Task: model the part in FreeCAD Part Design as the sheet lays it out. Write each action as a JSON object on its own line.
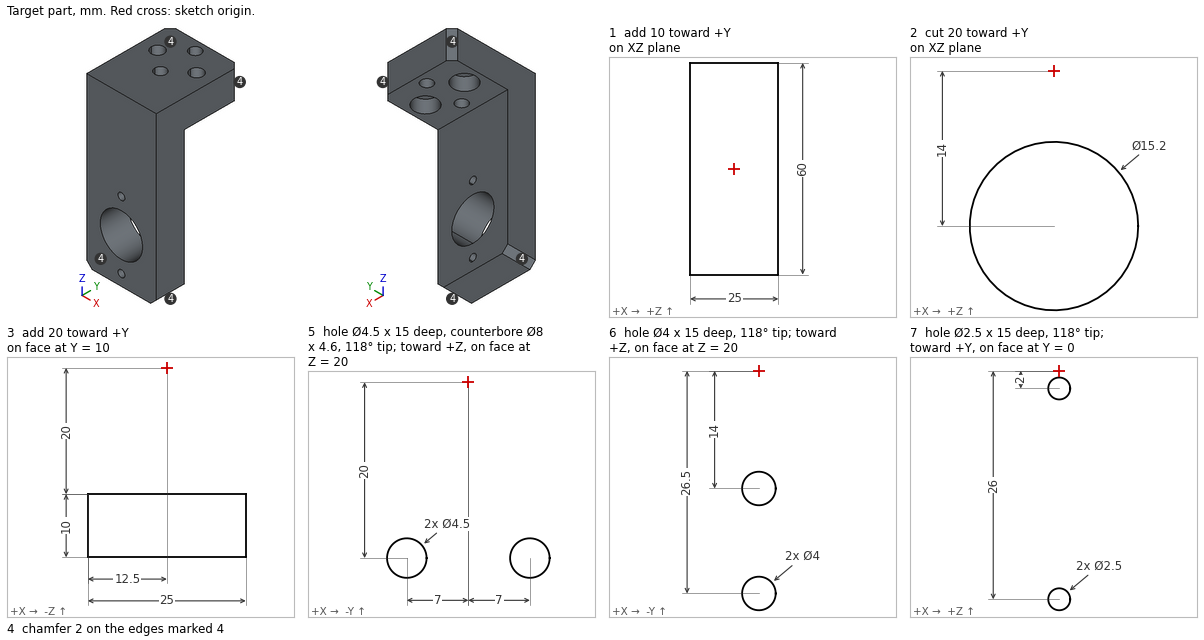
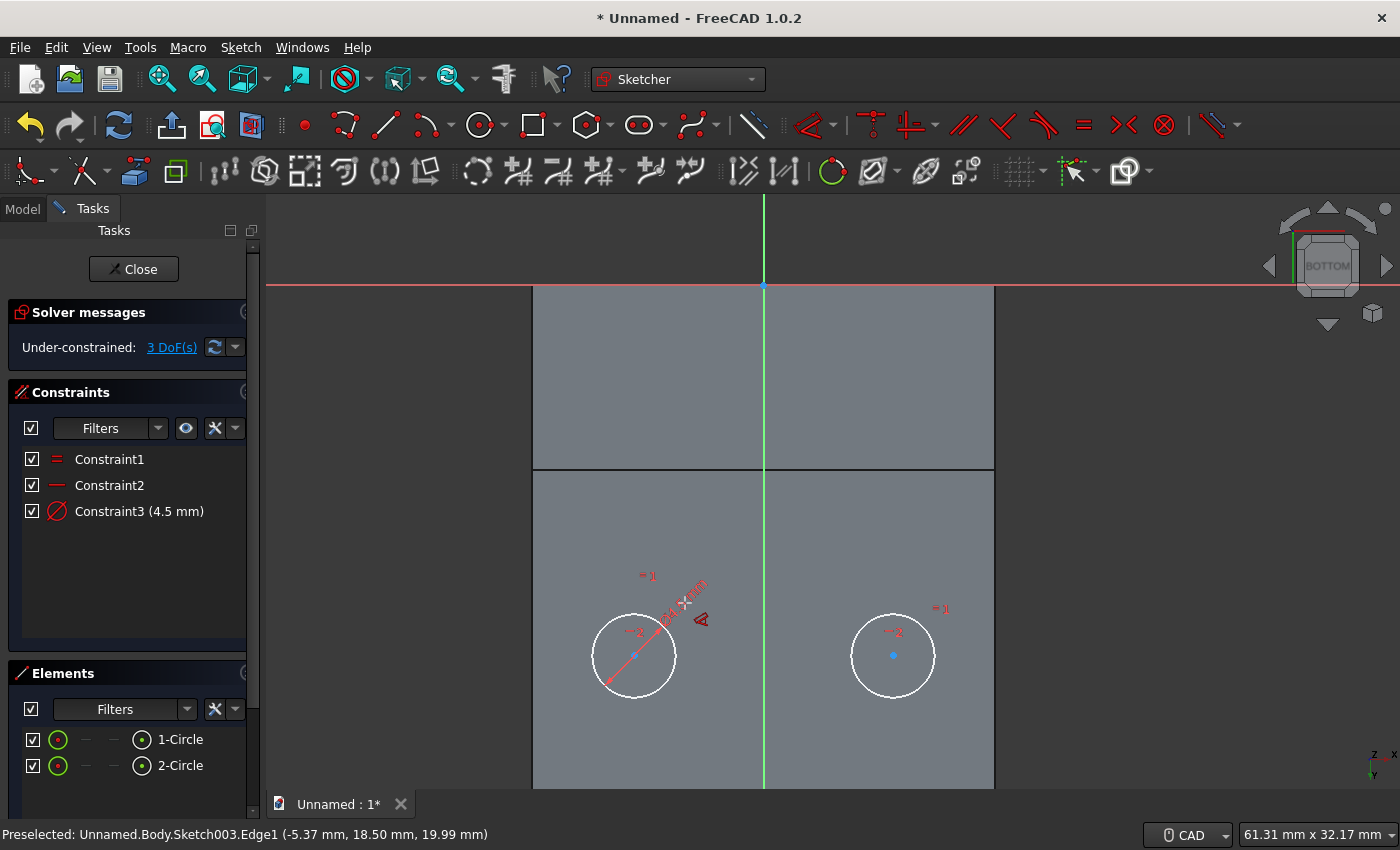
{"action": "left_click", "coordinate": [634, 656]}
{"action": "left_click", "coordinate": [699, 251]}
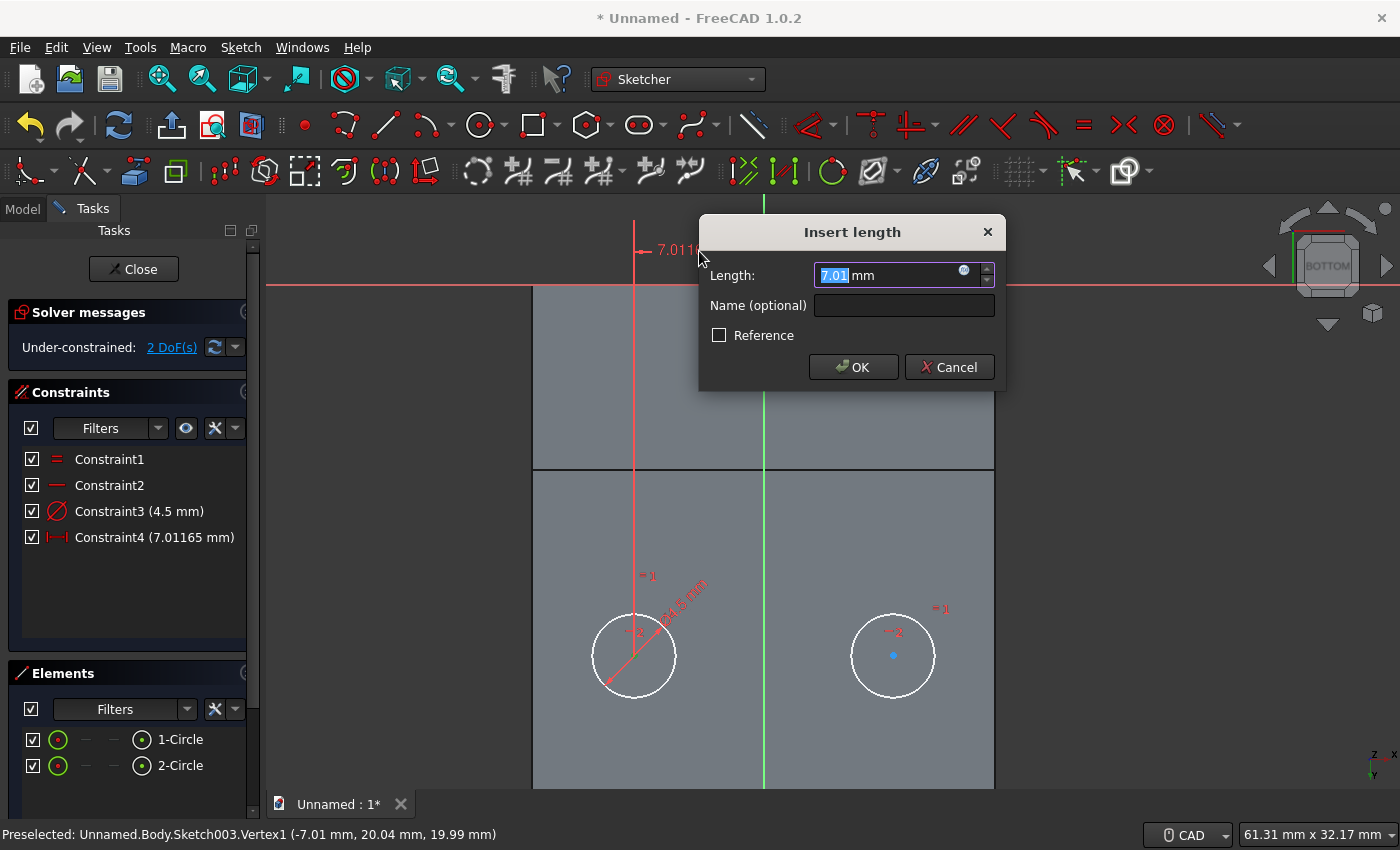
{"action": "type", "text": "7"}
{"action": "key", "text": "Return"}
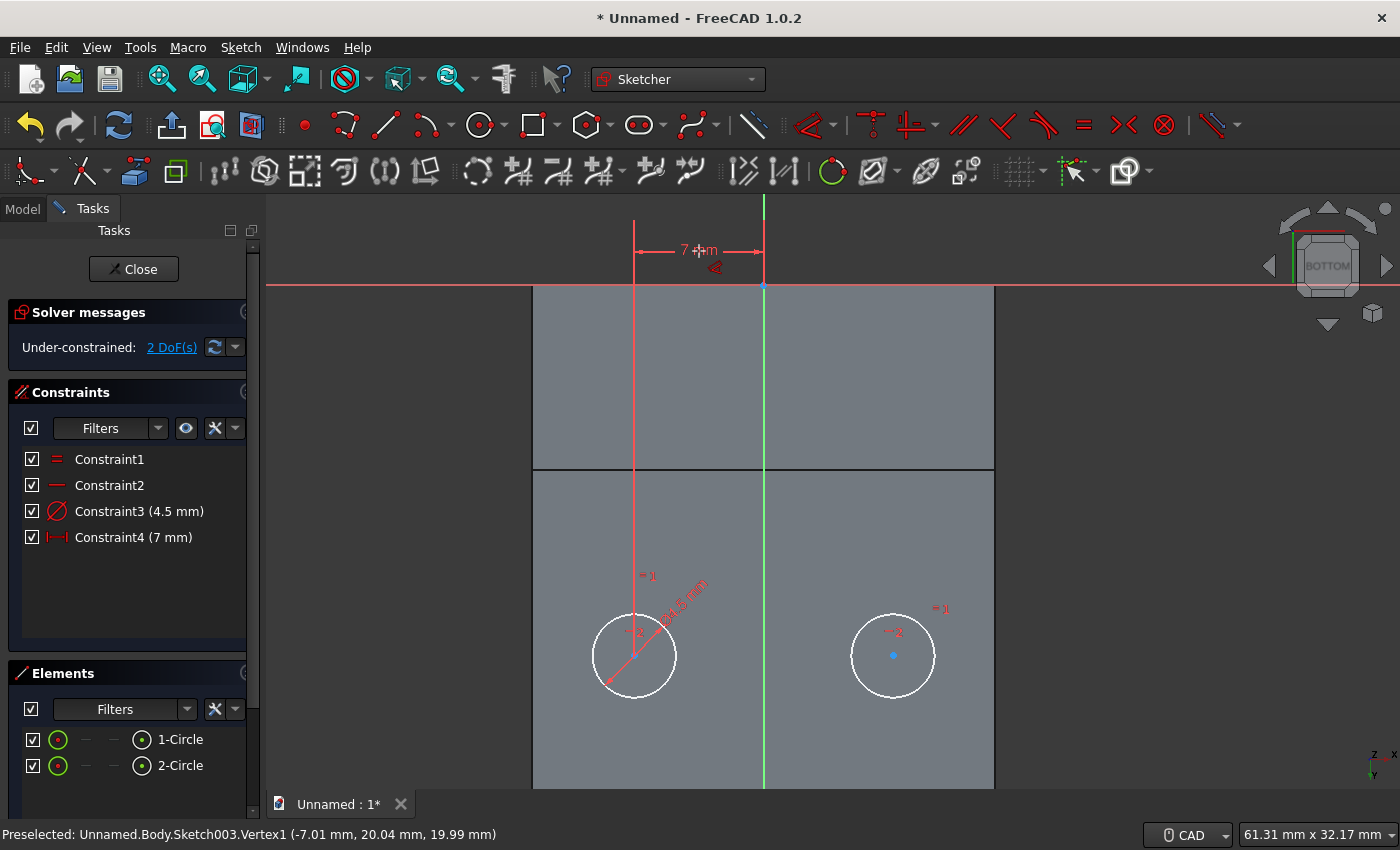
{"action": "left_click", "coordinate": [893, 656]}
{"action": "left_click", "coordinate": [828, 251]}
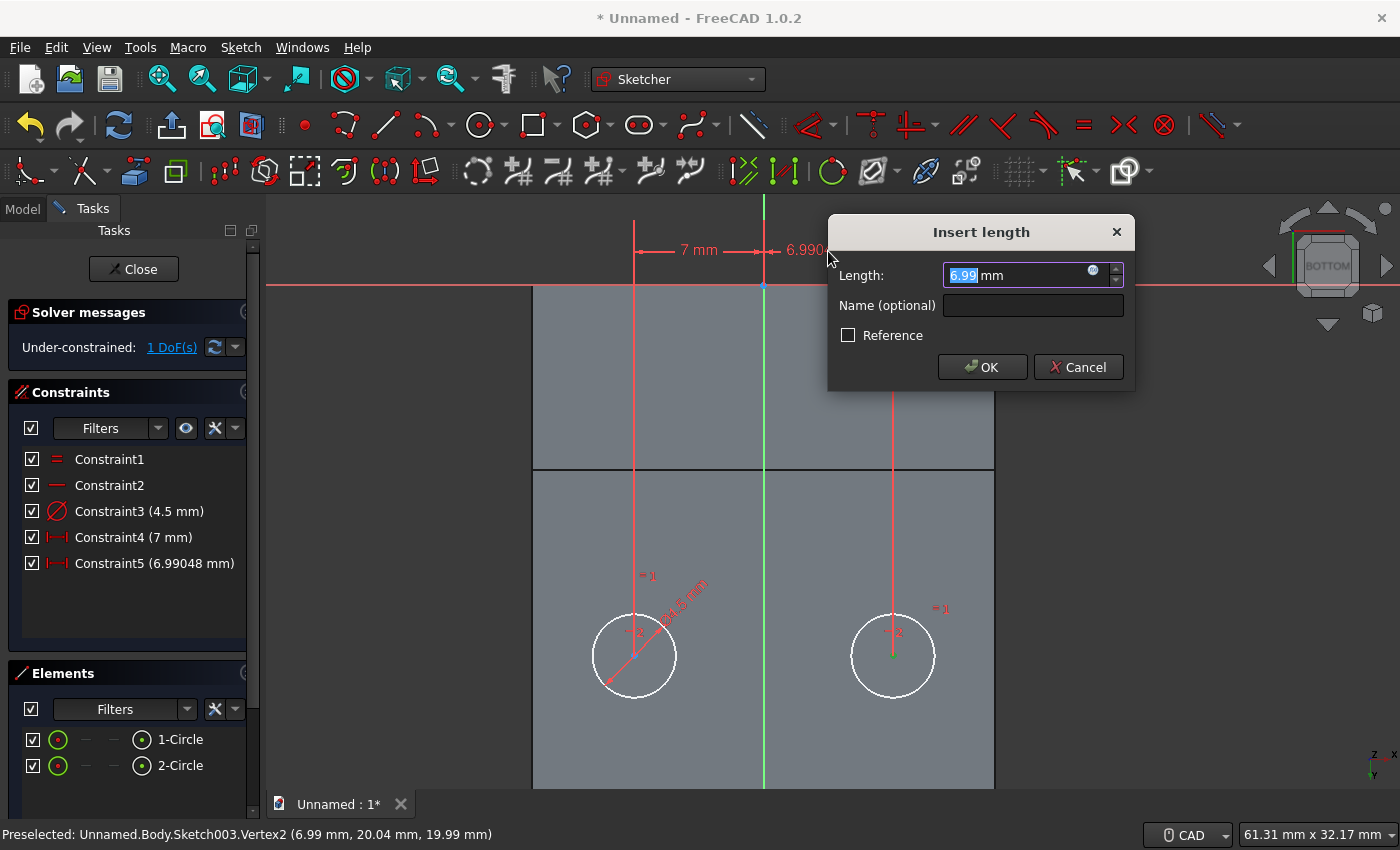
{"action": "type", "text": "7"}
{"action": "key", "text": "Return"}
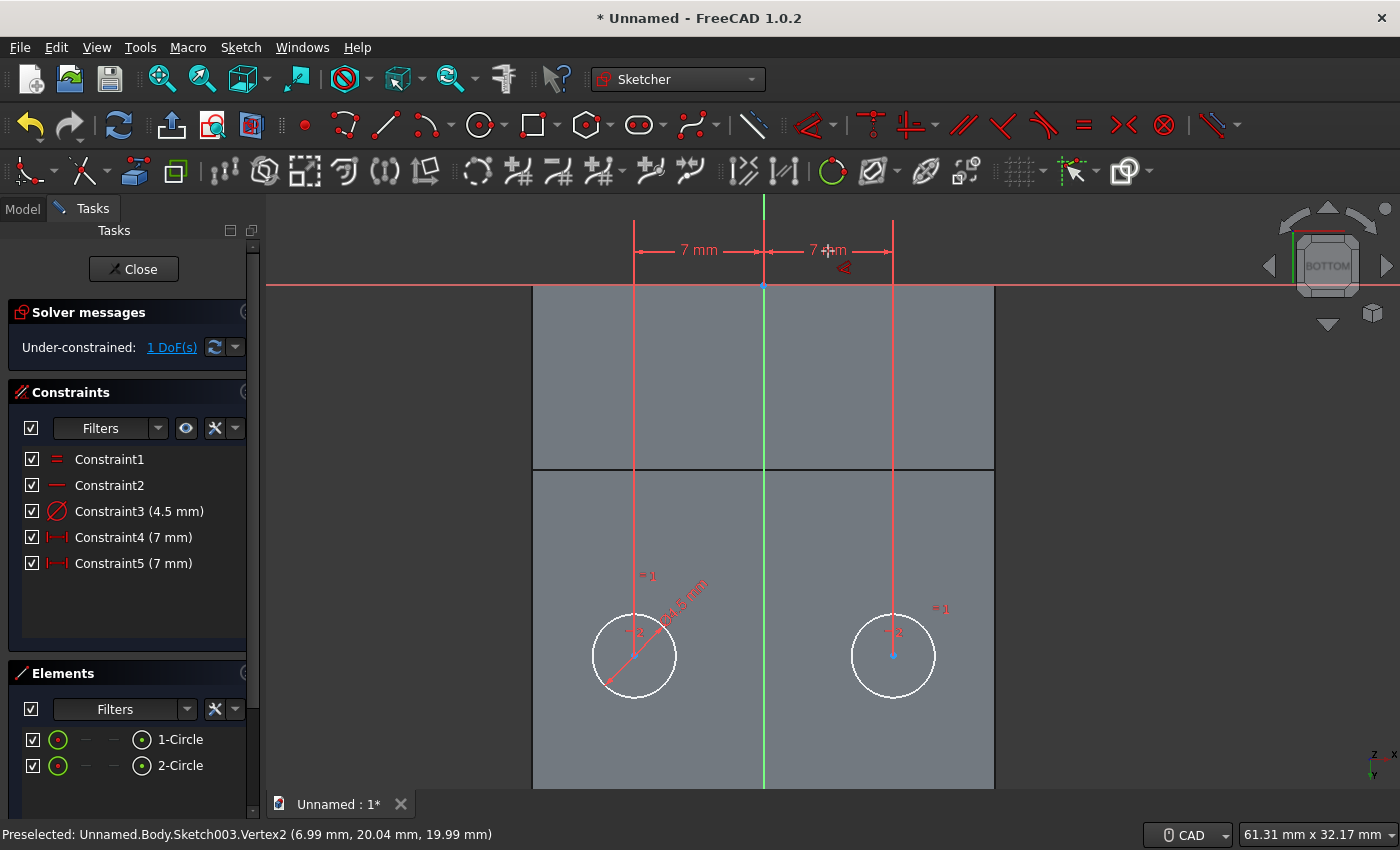
{"action": "left_click", "coordinate": [634, 656]}
{"action": "left_click", "coordinate": [600, 471]}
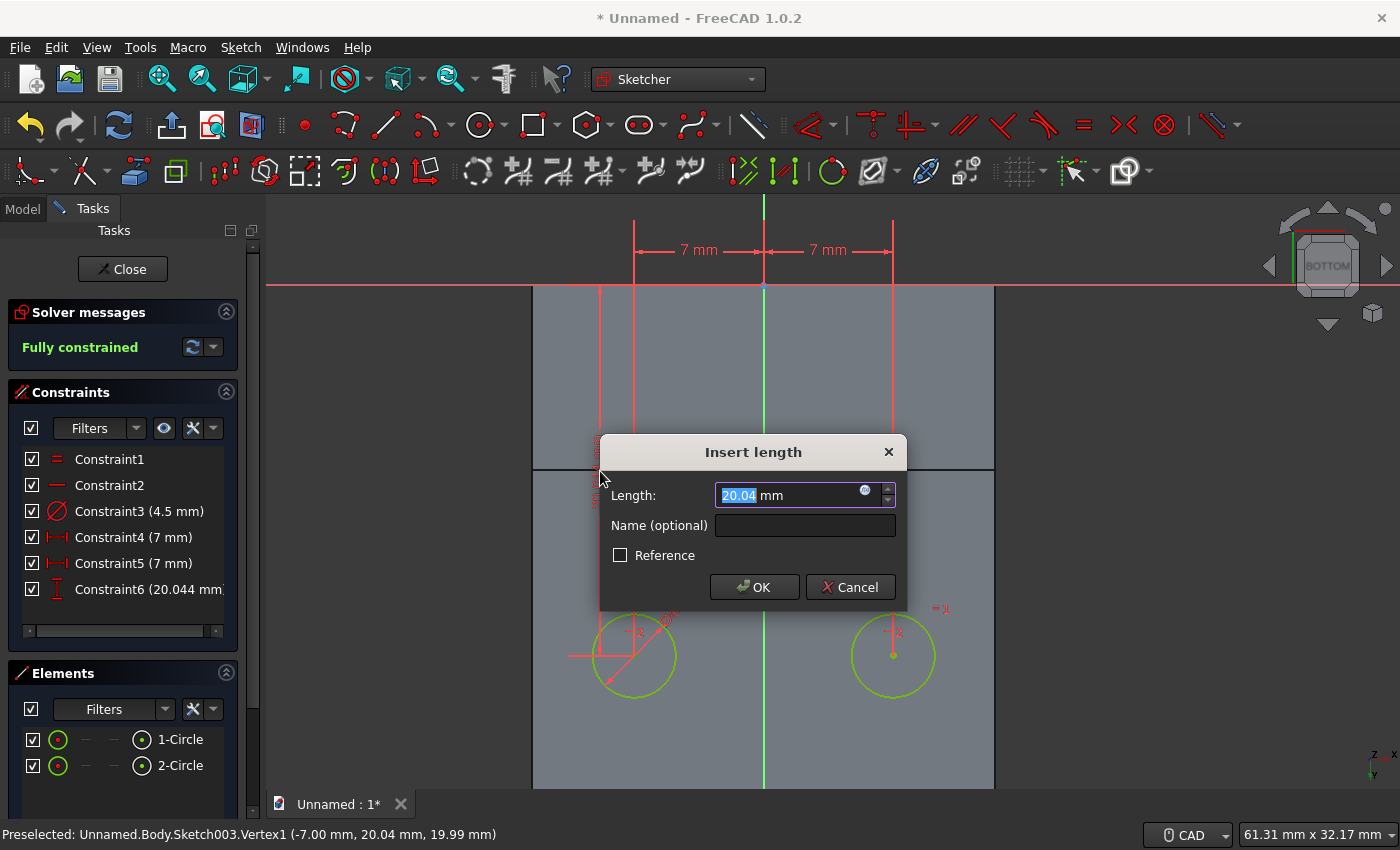
{"action": "type", "text": "20"}
{"action": "key", "text": "Return"}
{"action": "key", "text": "Escape"}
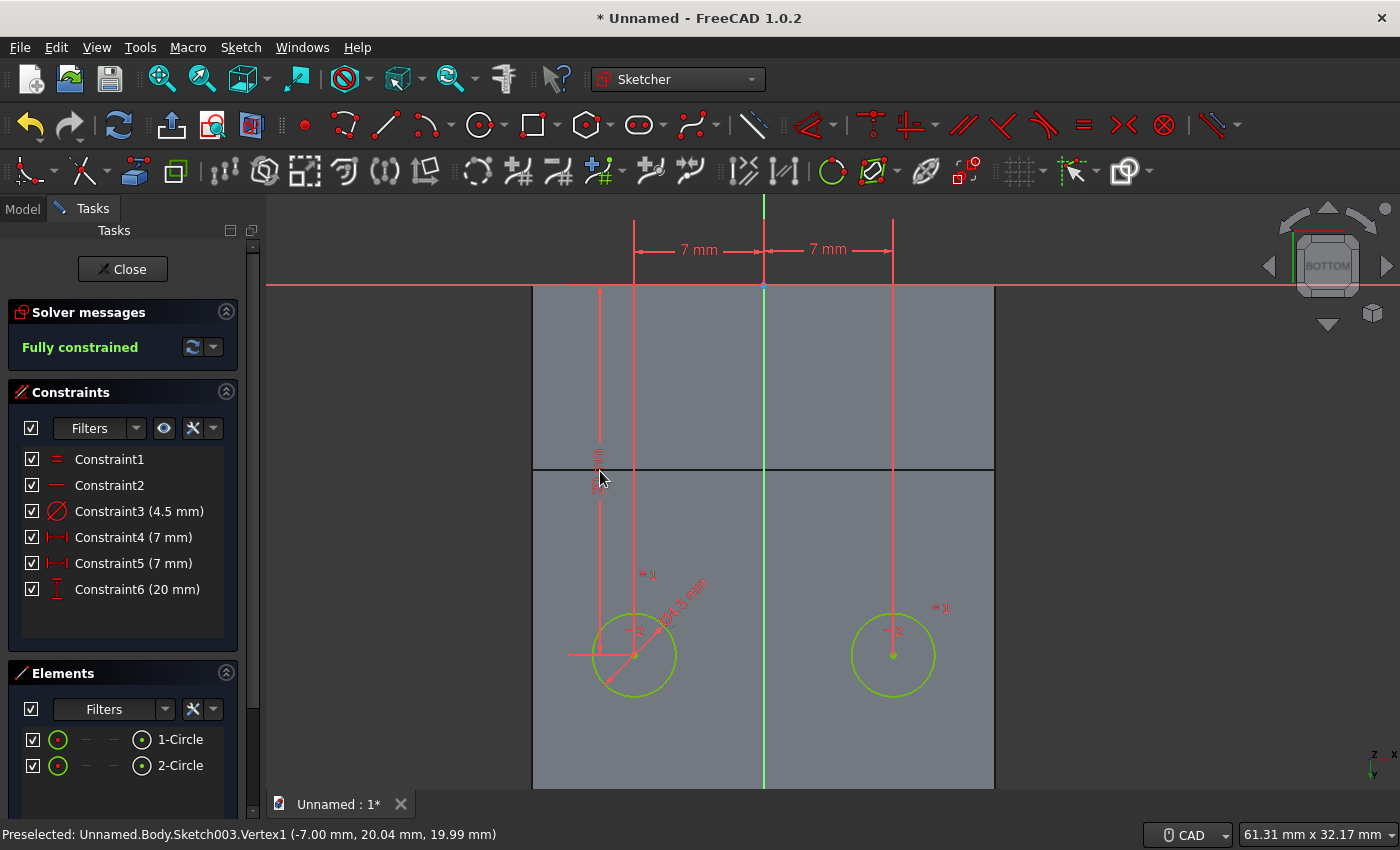
{"action": "left_click", "coordinate": [123, 269]}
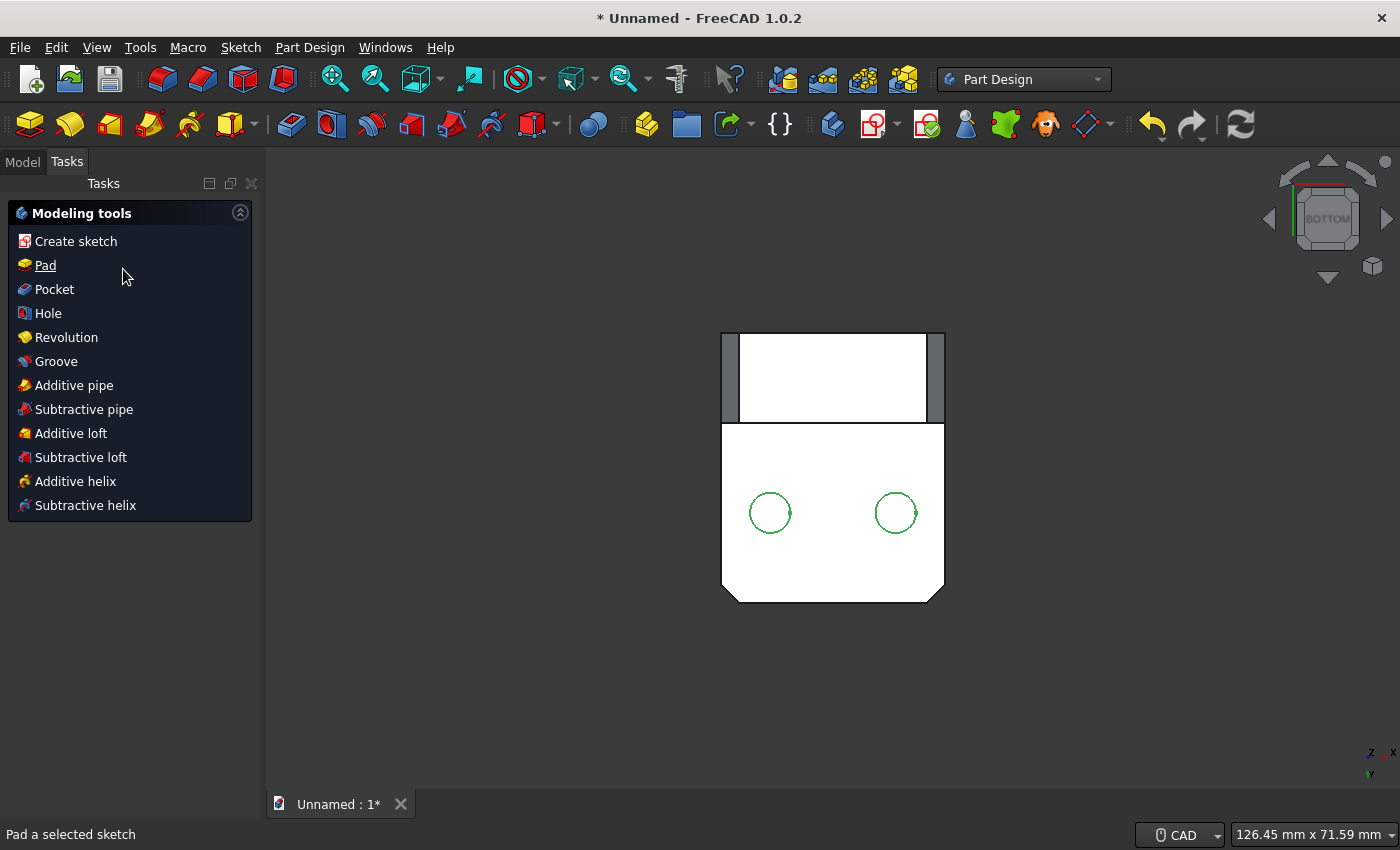
{"action": "left_click", "coordinate": [332, 124]}